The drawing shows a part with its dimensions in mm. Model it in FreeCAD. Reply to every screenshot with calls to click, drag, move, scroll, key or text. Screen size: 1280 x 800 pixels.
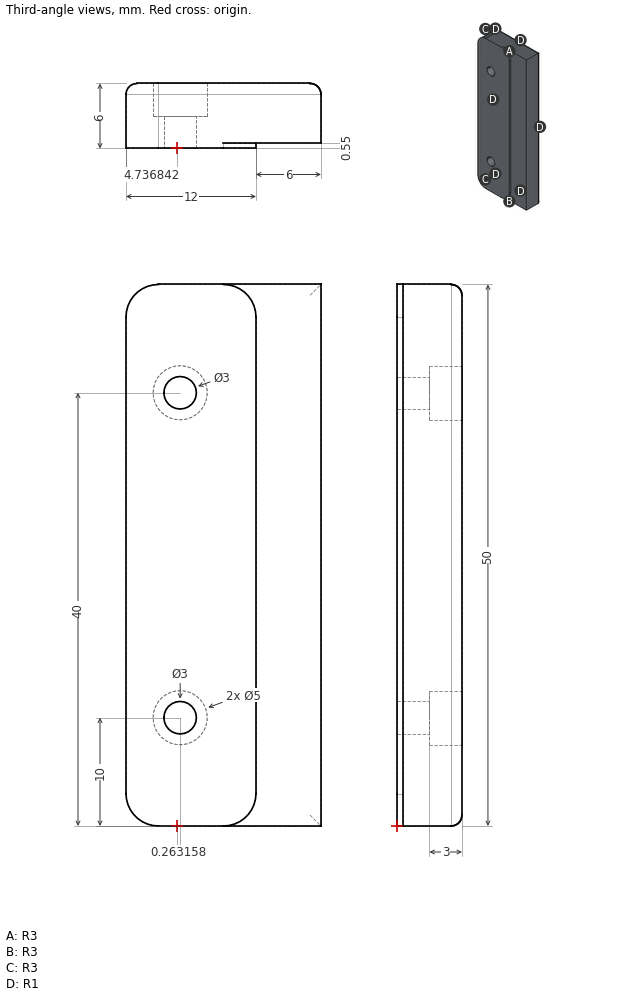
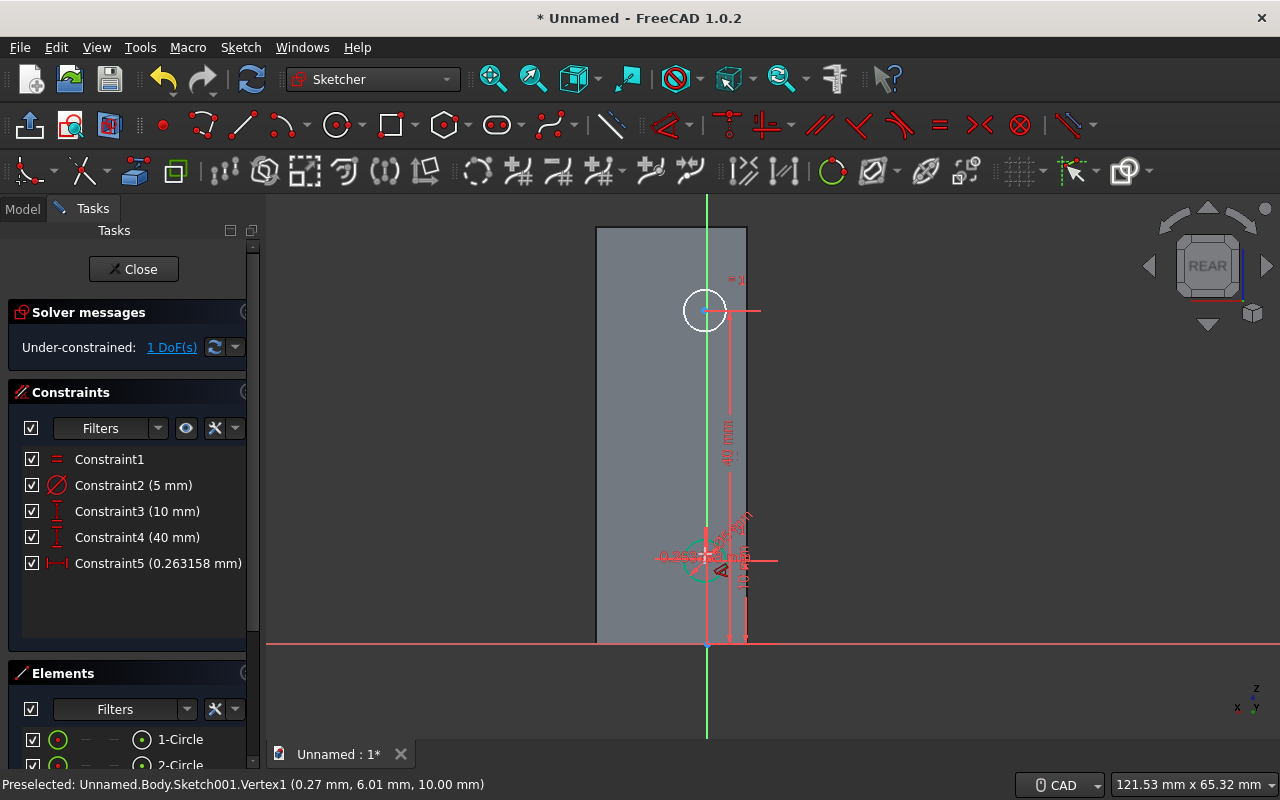
scroll(705, 311, up, 15)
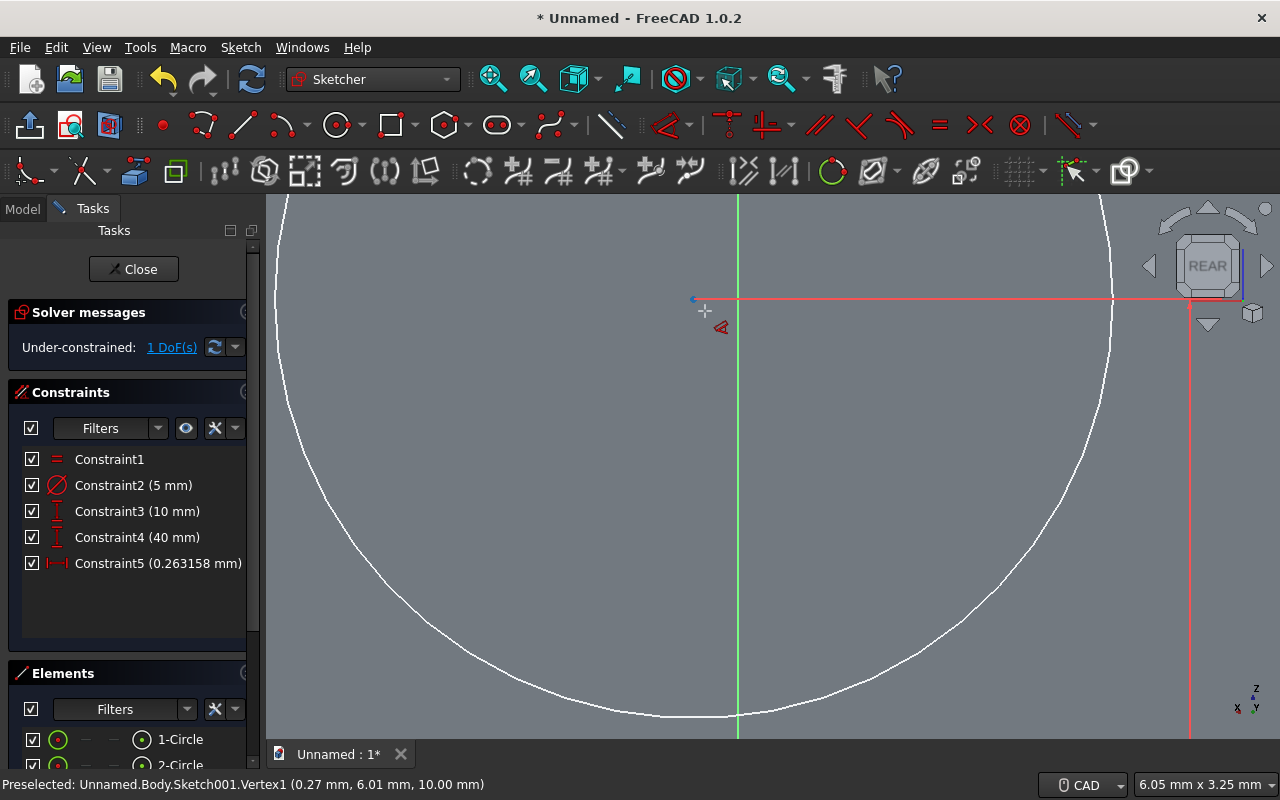
click(694, 299)
click(716, 265)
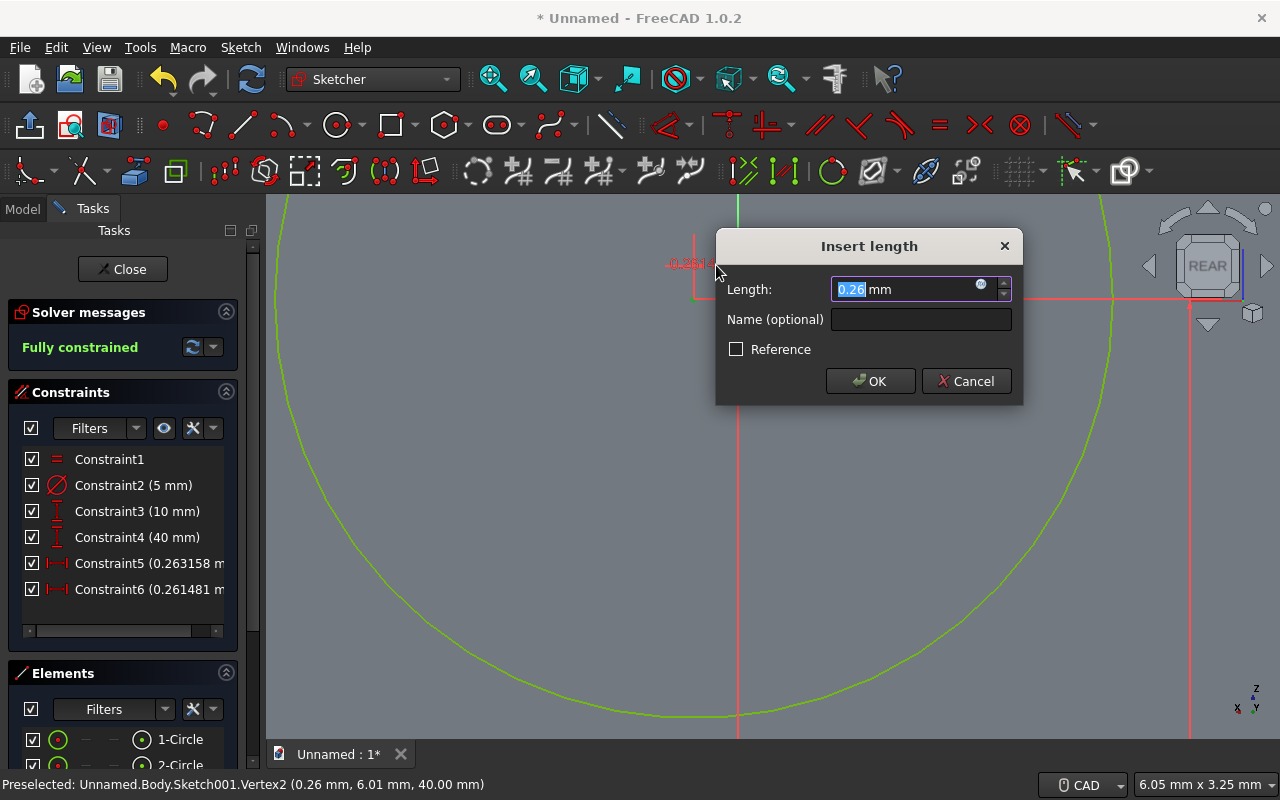
text(0.263158)
key(Return)
key(Escape)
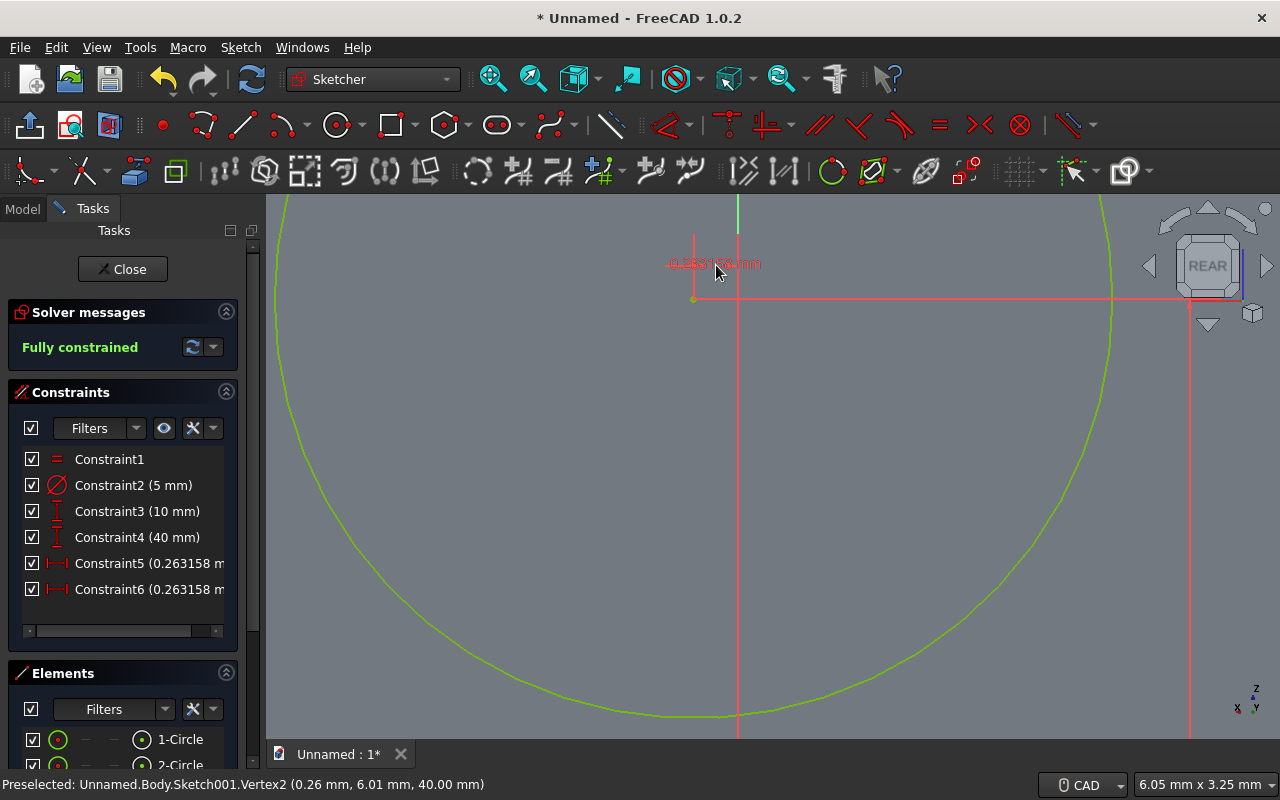
click(123, 269)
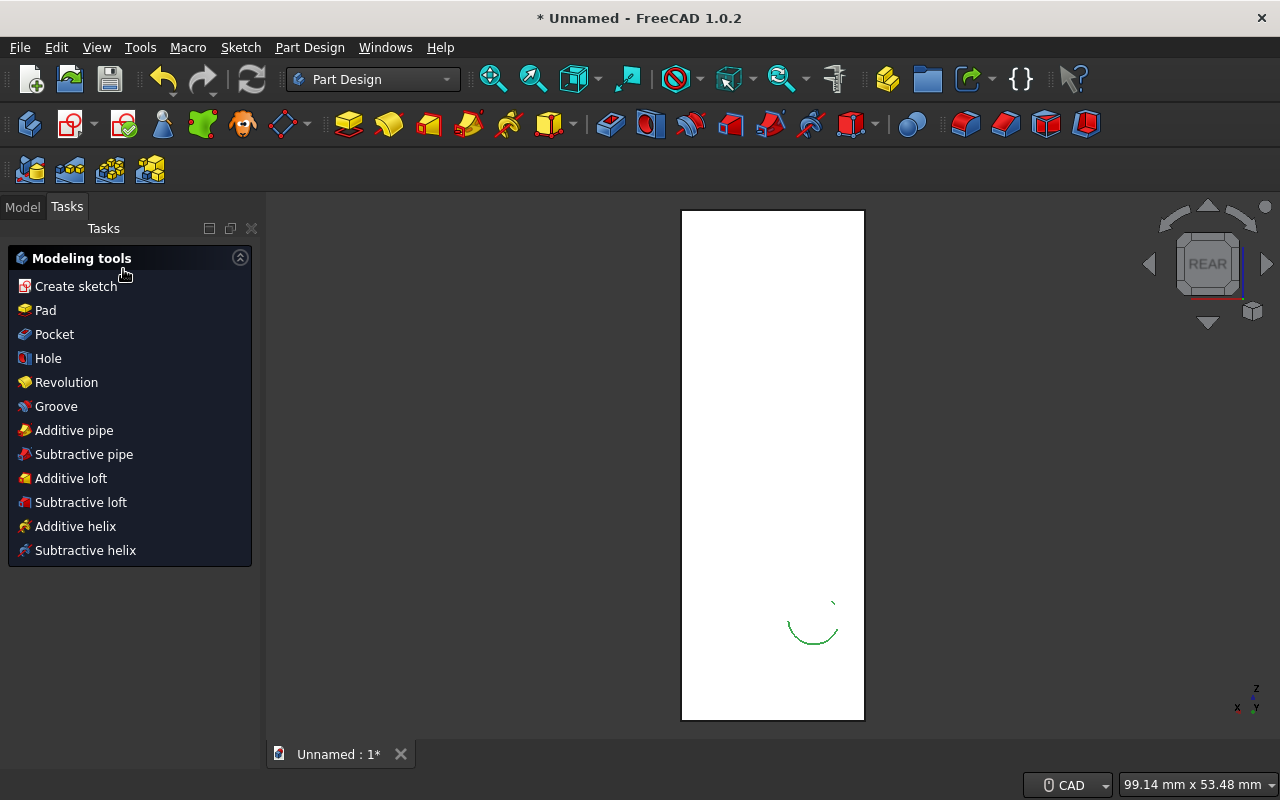
click(612, 124)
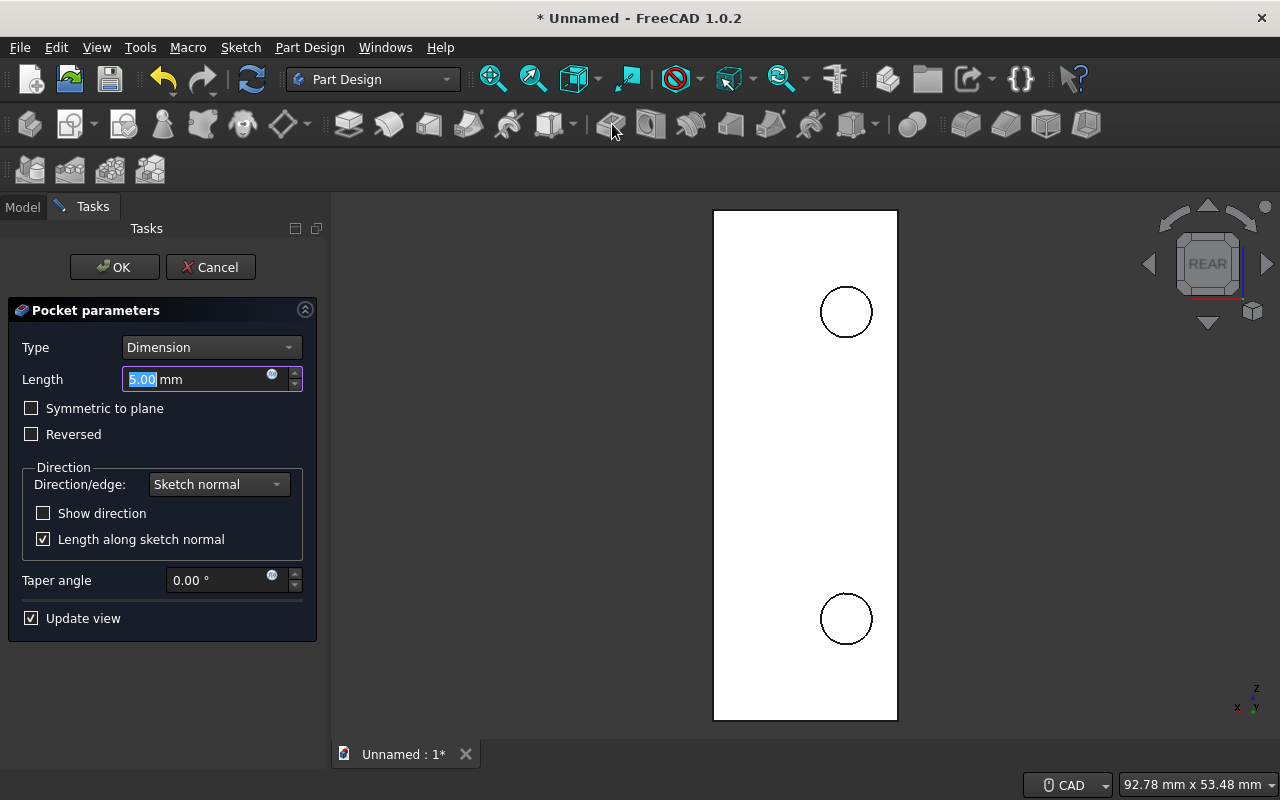
text(3)
key(Tab)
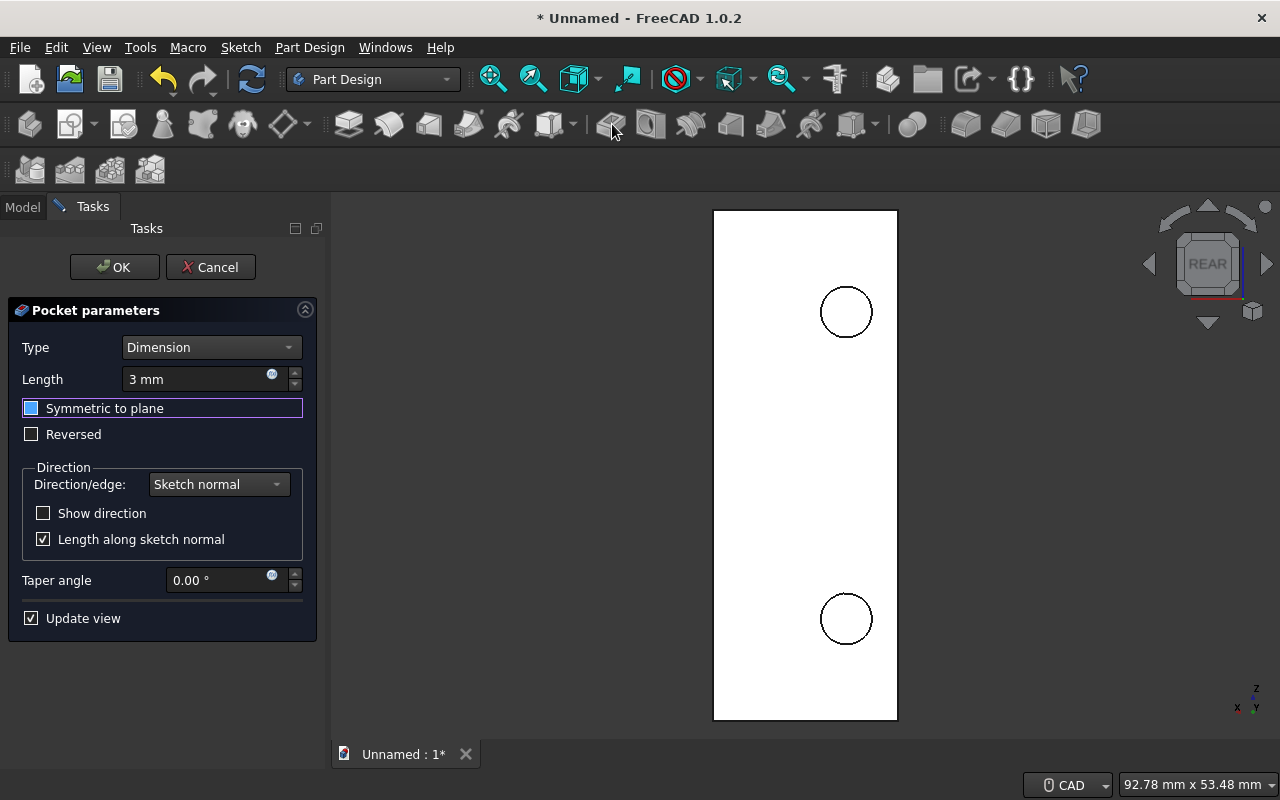
click(115, 267)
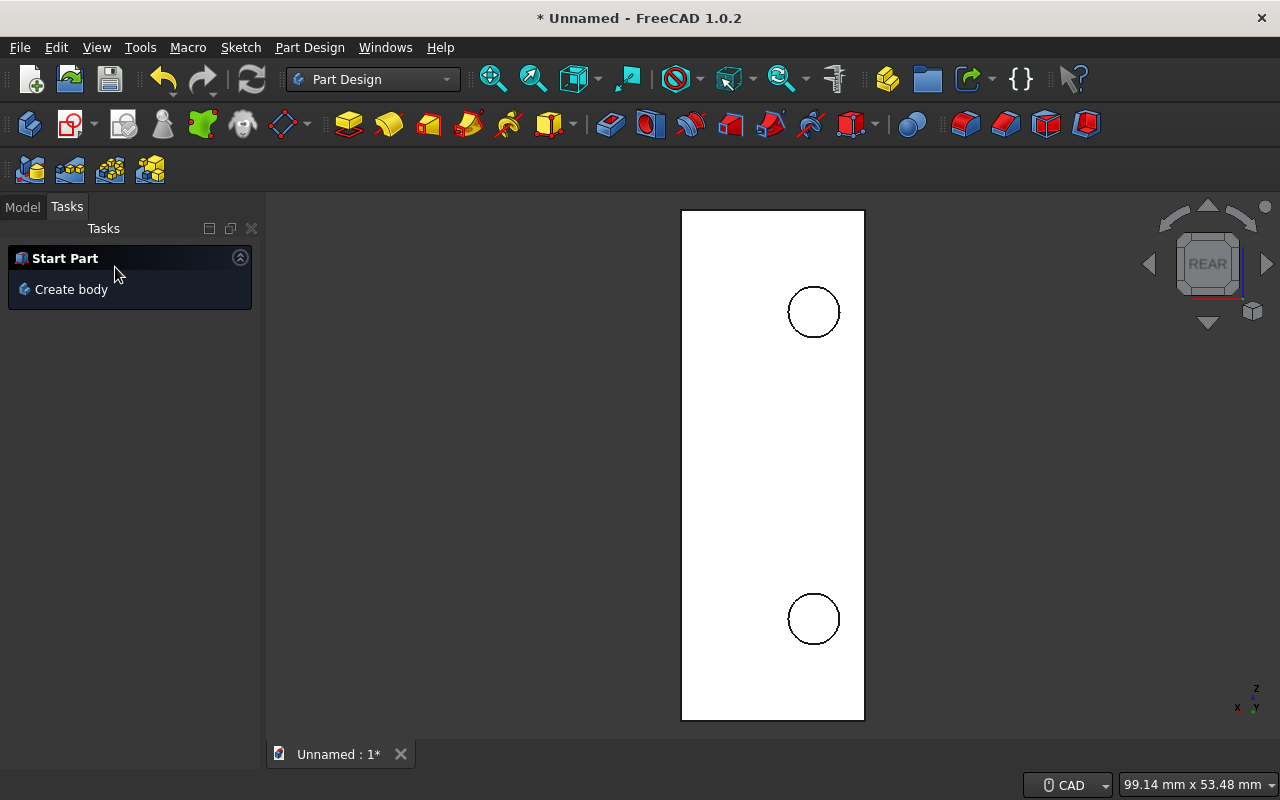
click(814, 311)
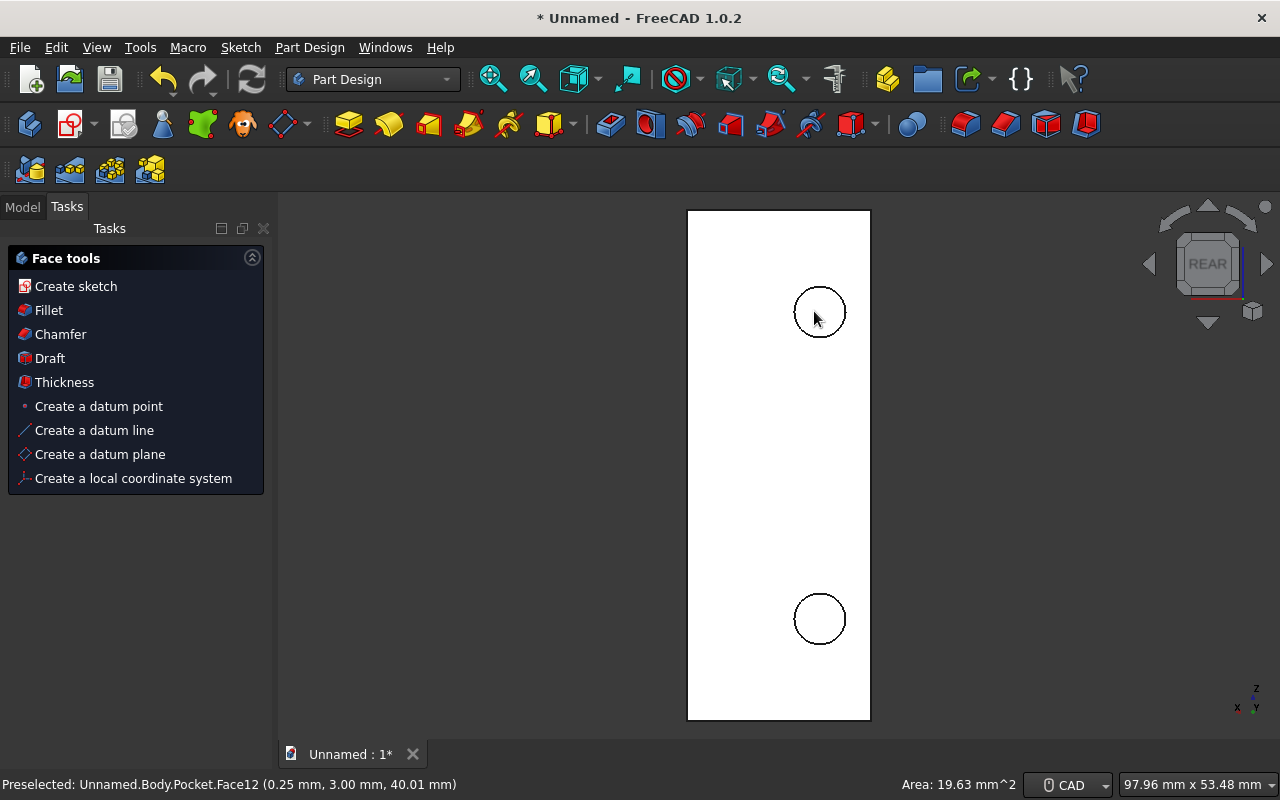
click(70, 124)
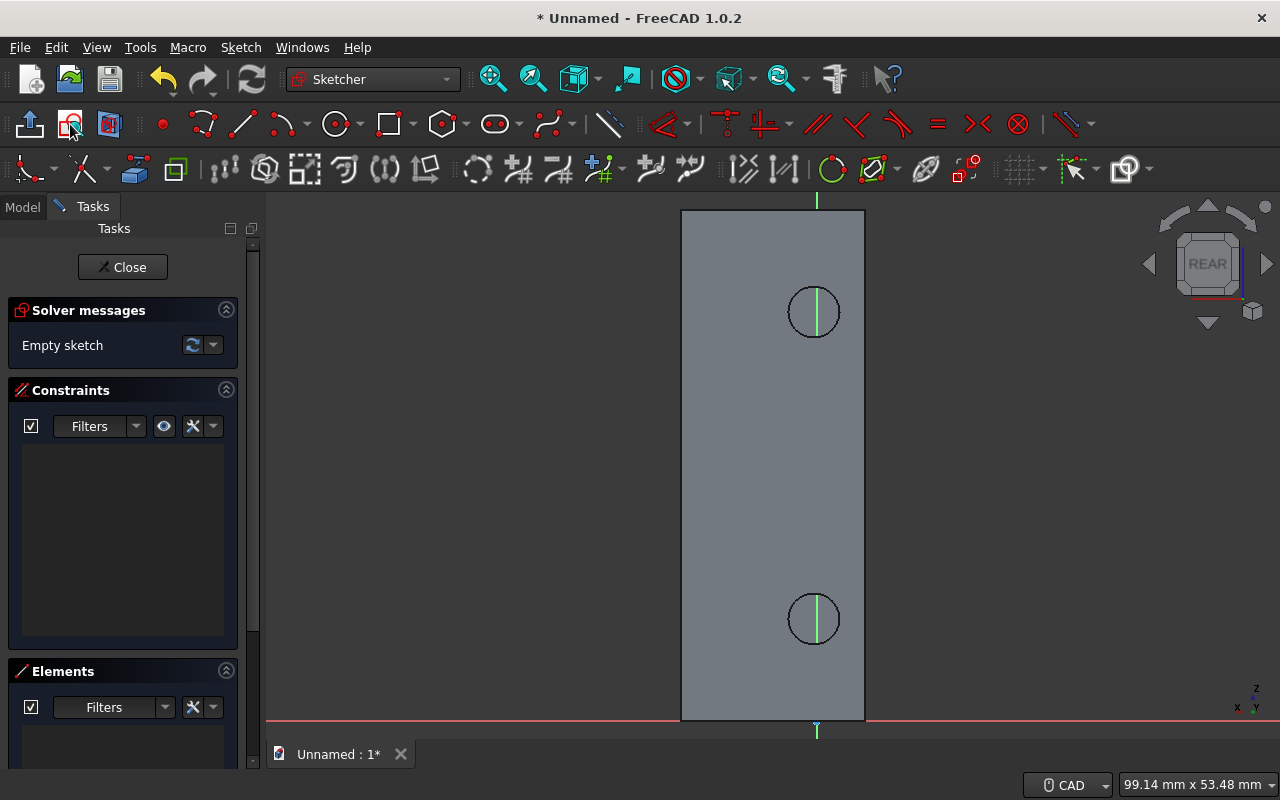
scroll(825, 297, up, 12)